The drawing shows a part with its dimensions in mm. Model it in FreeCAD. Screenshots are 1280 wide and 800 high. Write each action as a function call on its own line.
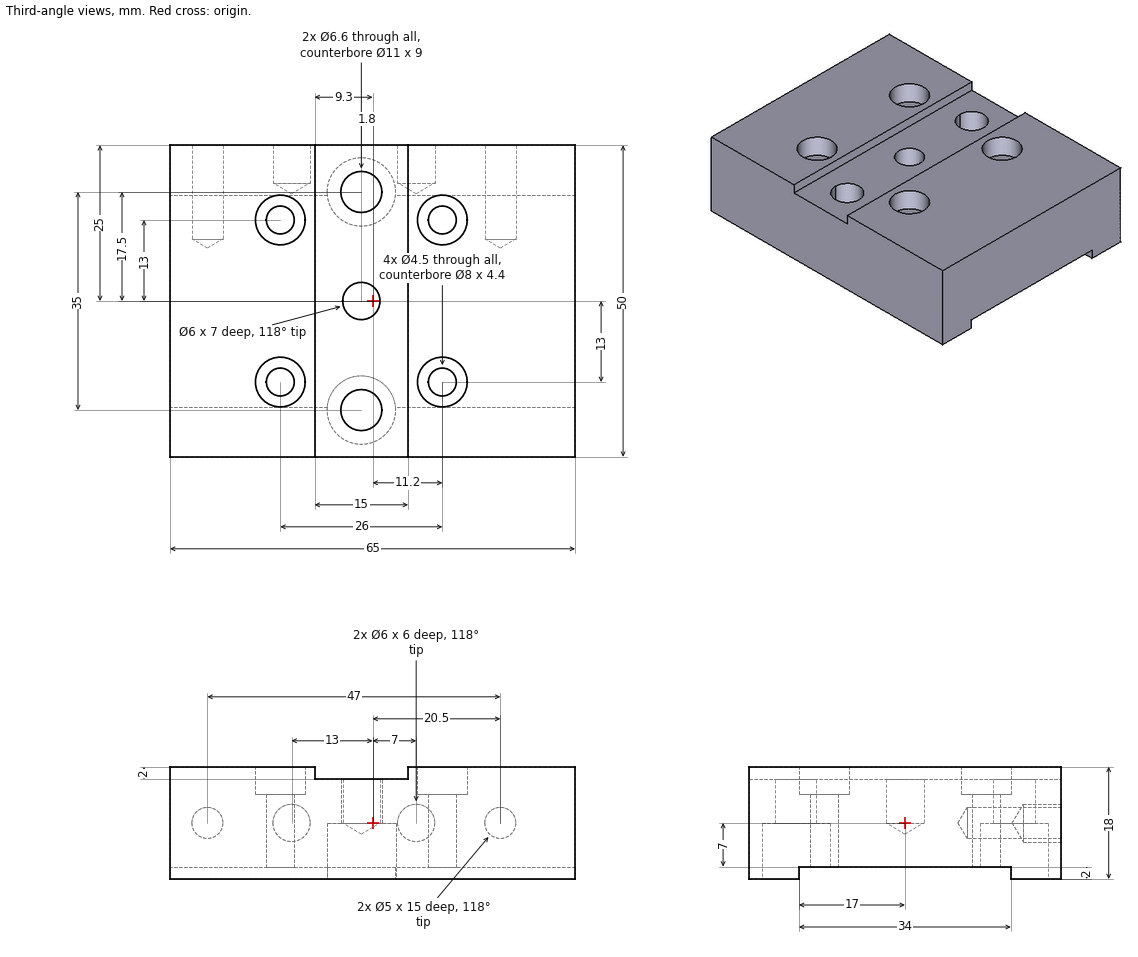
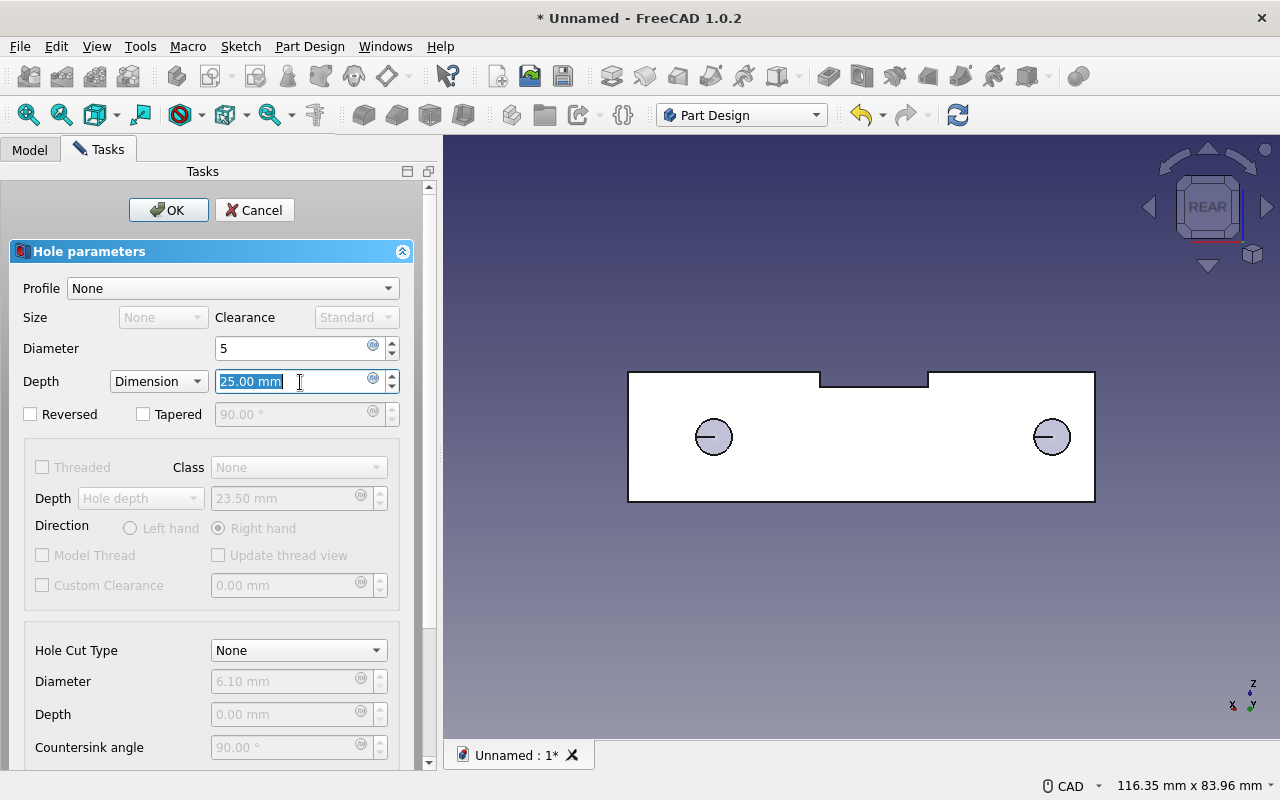
text(15)
key(Tab)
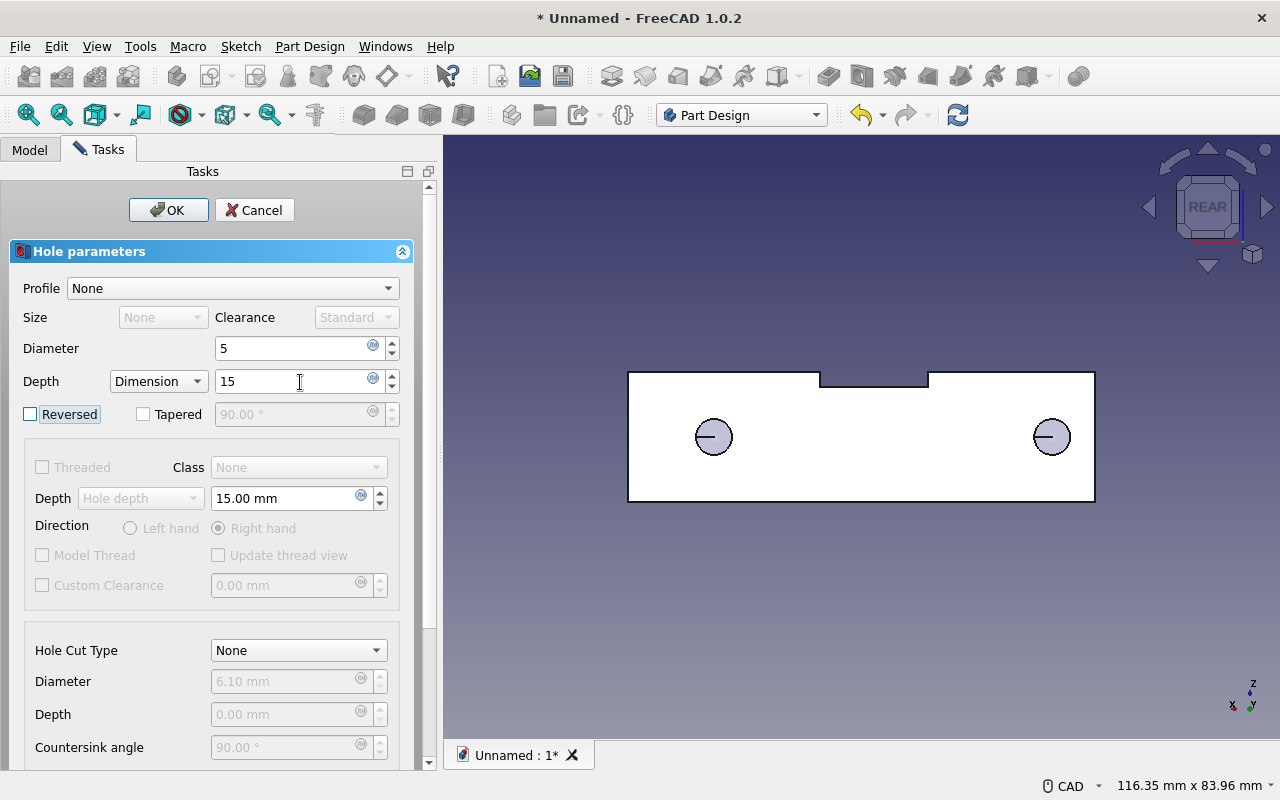
click(169, 210)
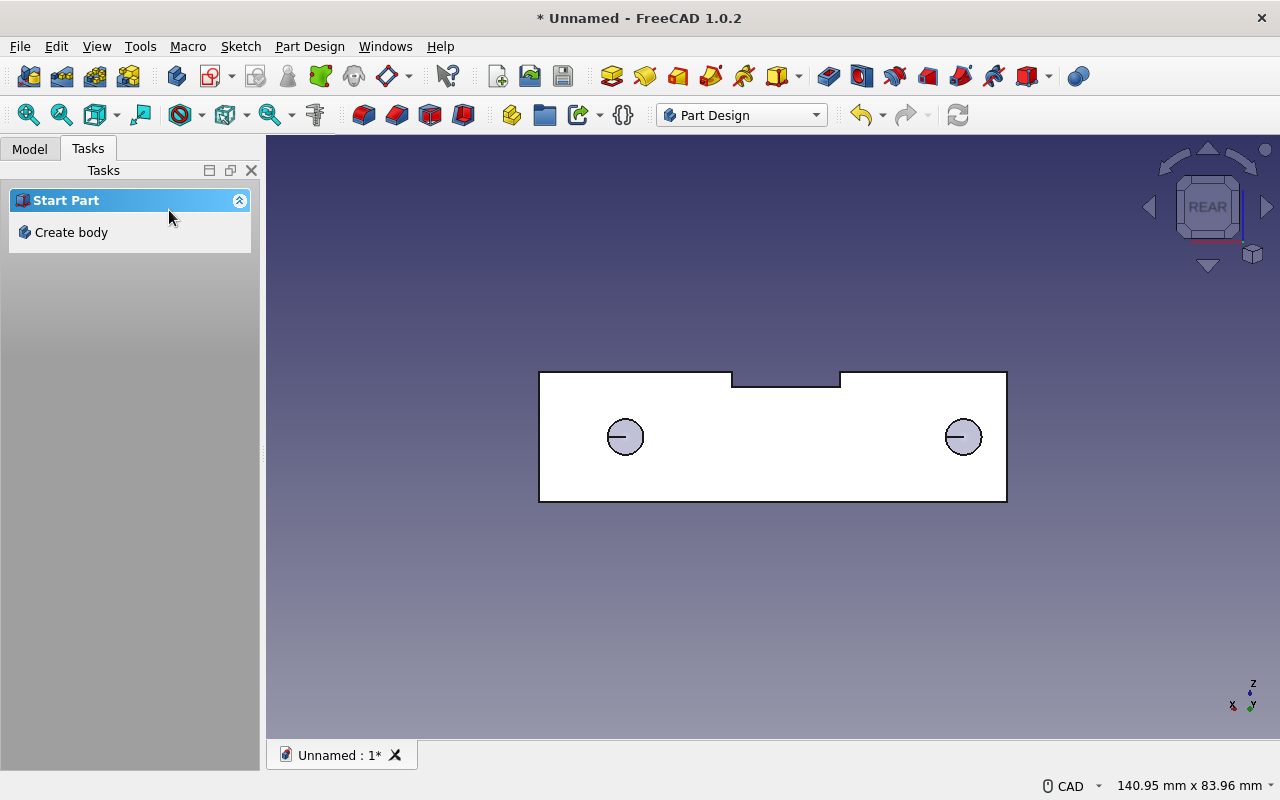
click(706, 436)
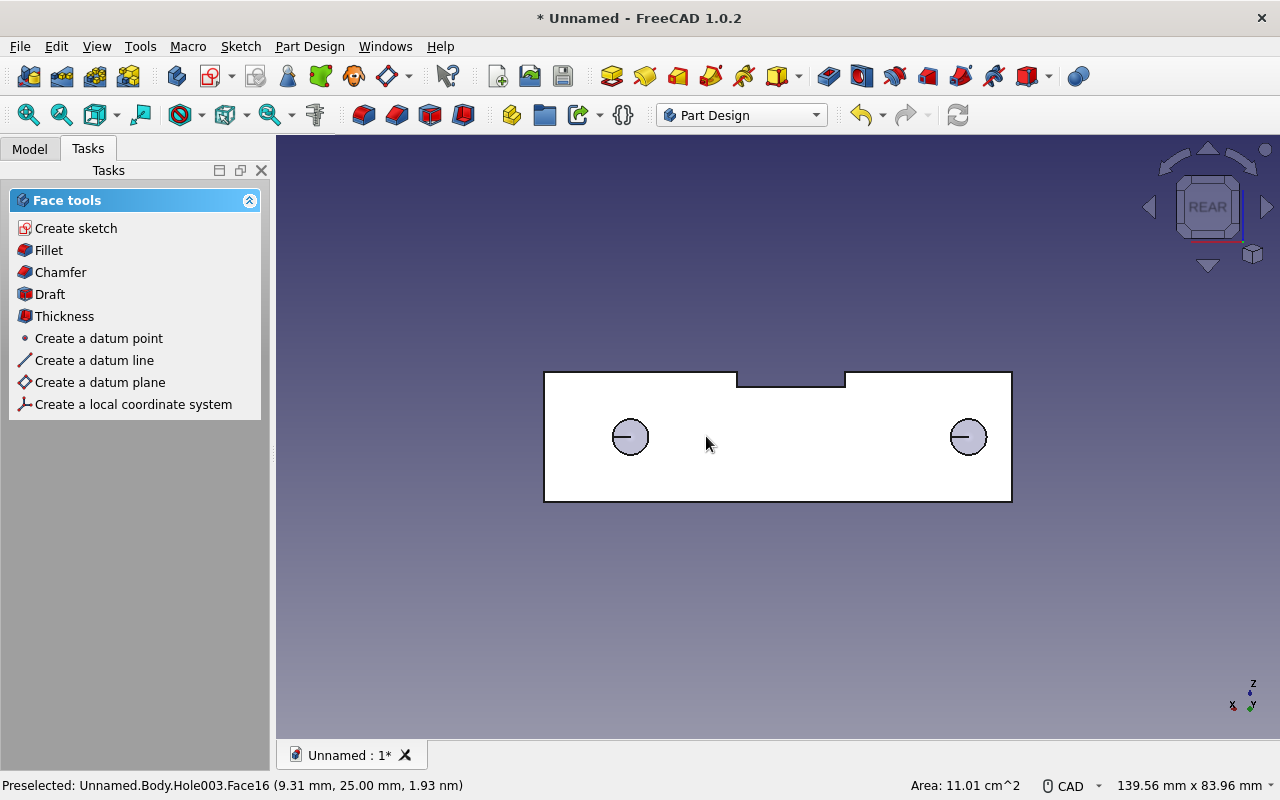
click(210, 76)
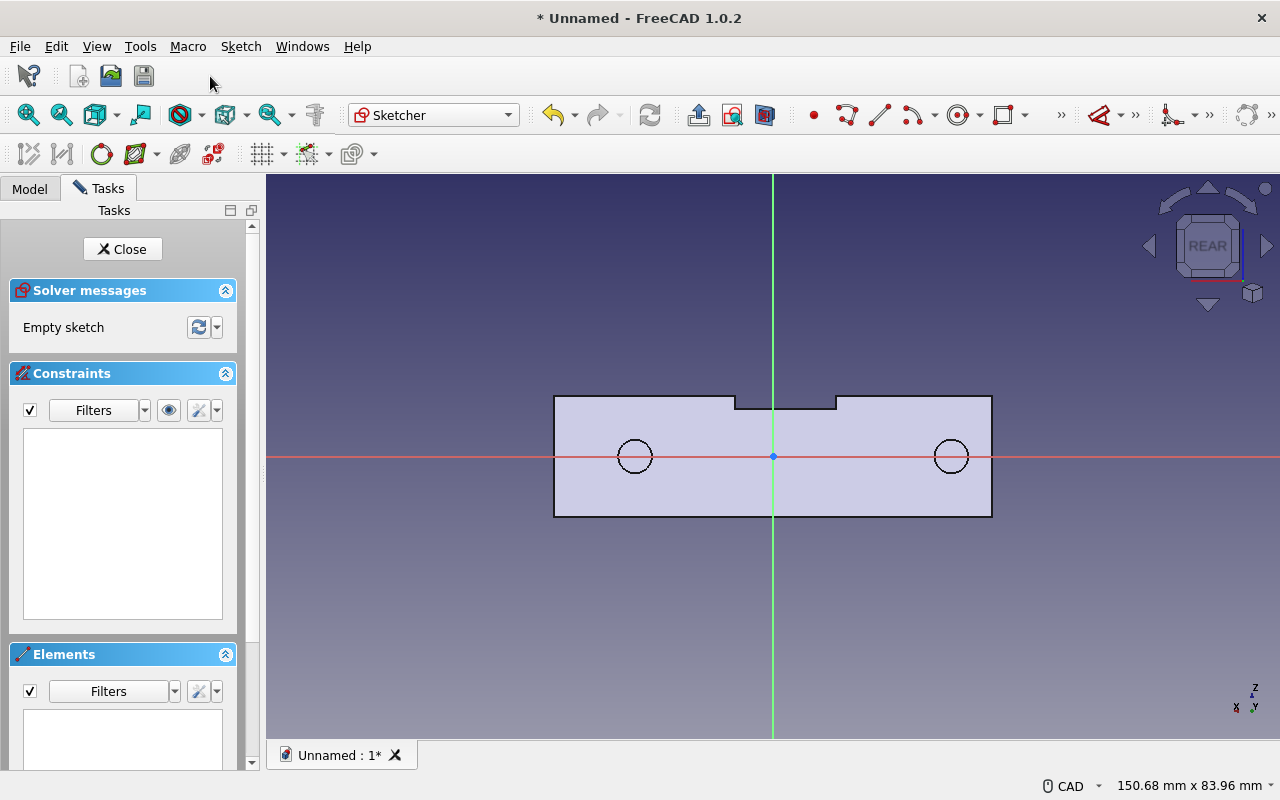
scroll(831, 457, up, 6)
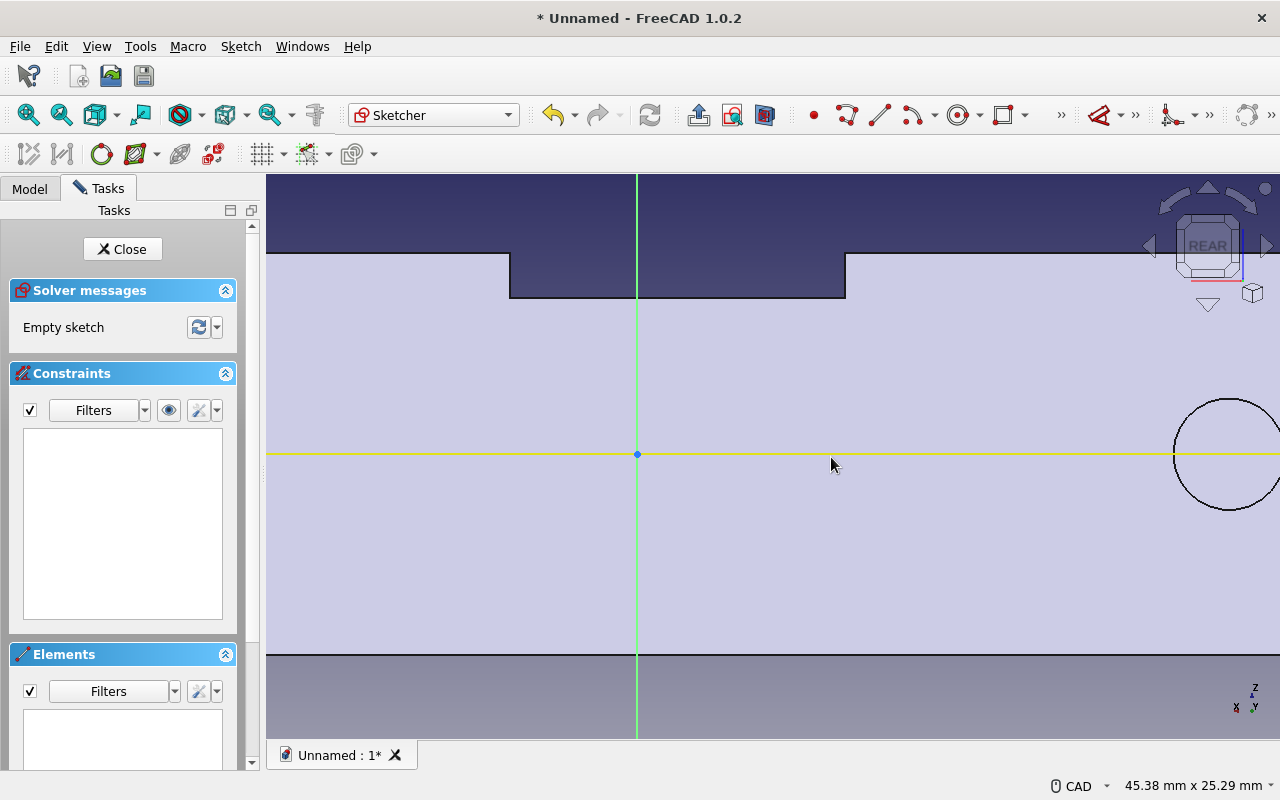
key(g)
key(c)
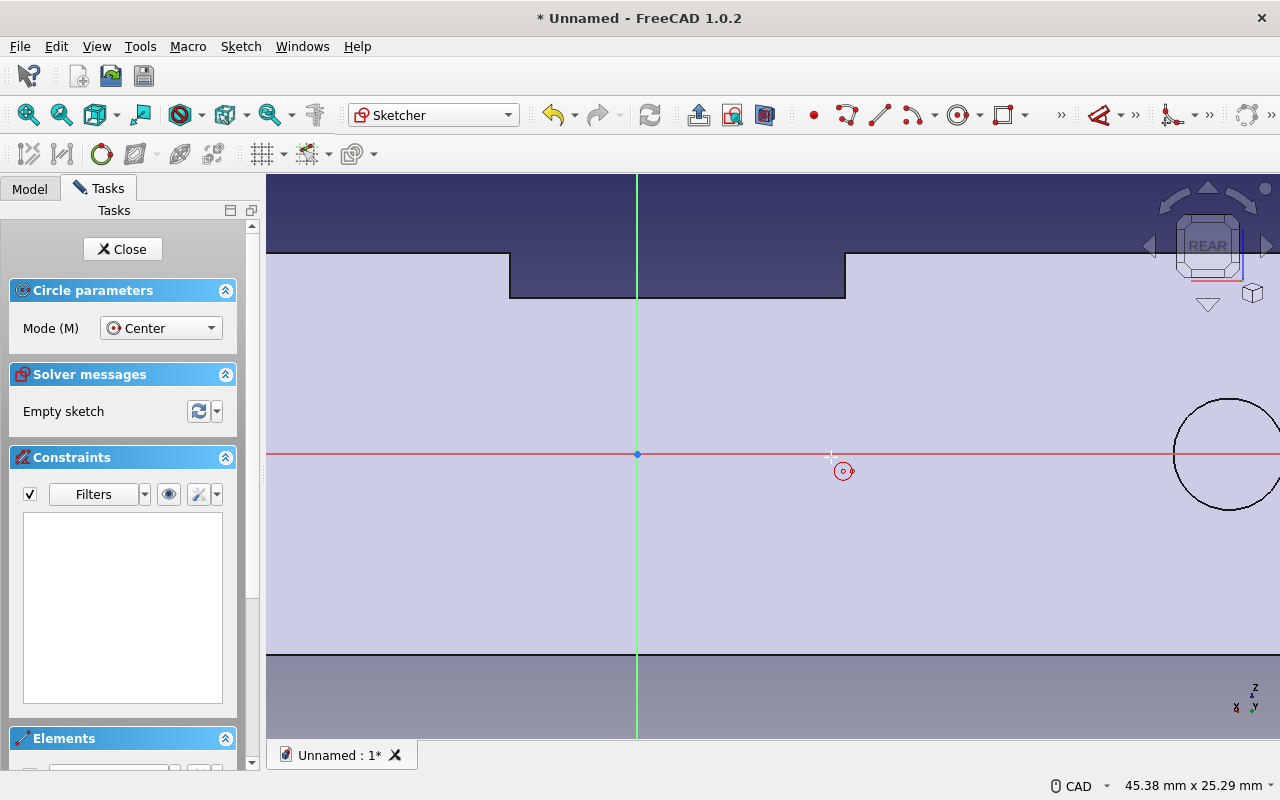
click(481, 454)
move(528, 407)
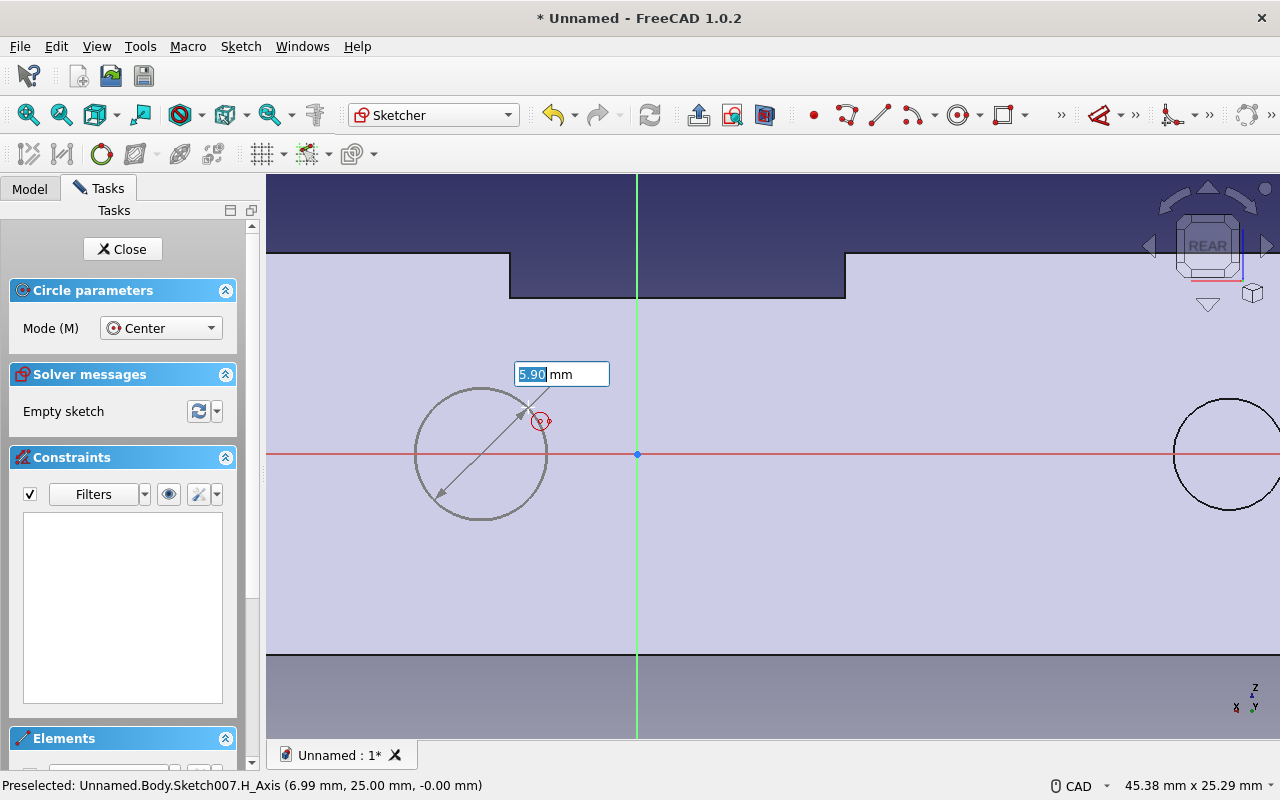
text(6)
key(Return)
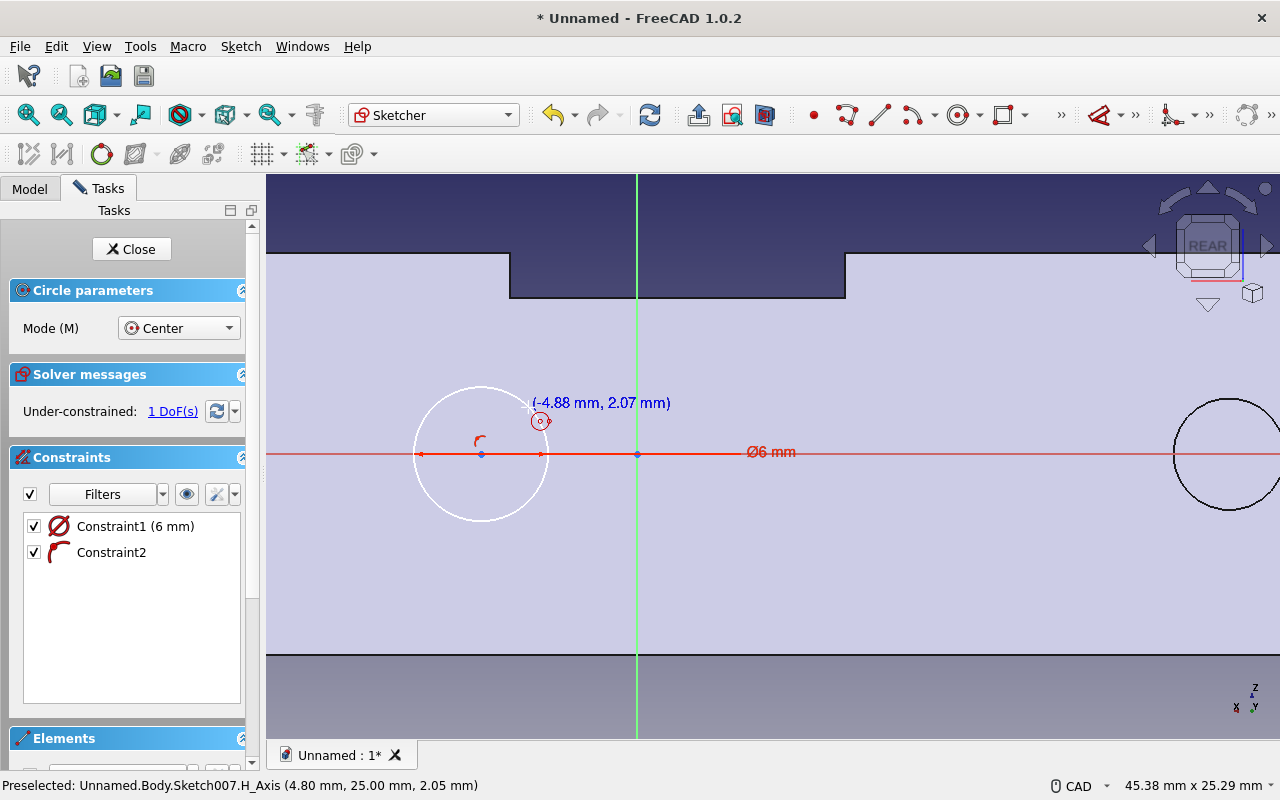
click(928, 454)
move(975, 407)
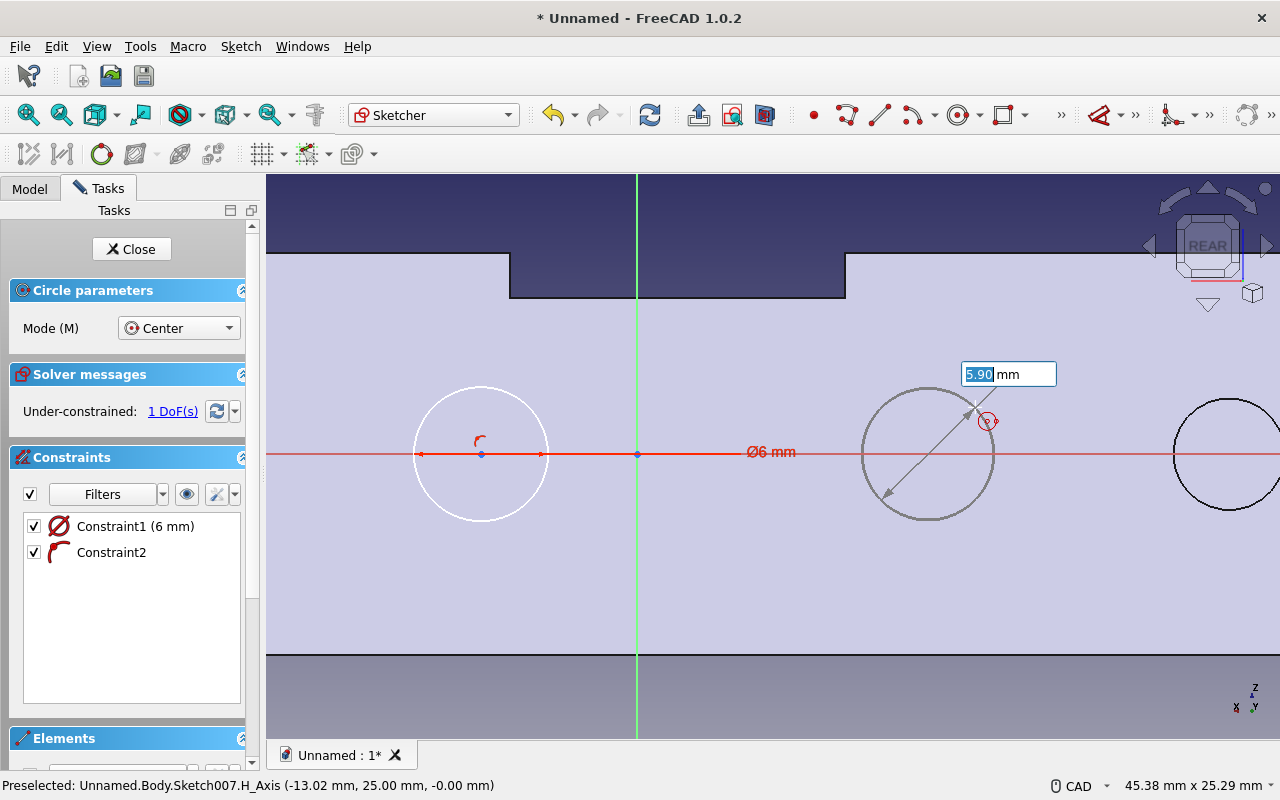
text(6)
key(Return)
key(Escape)